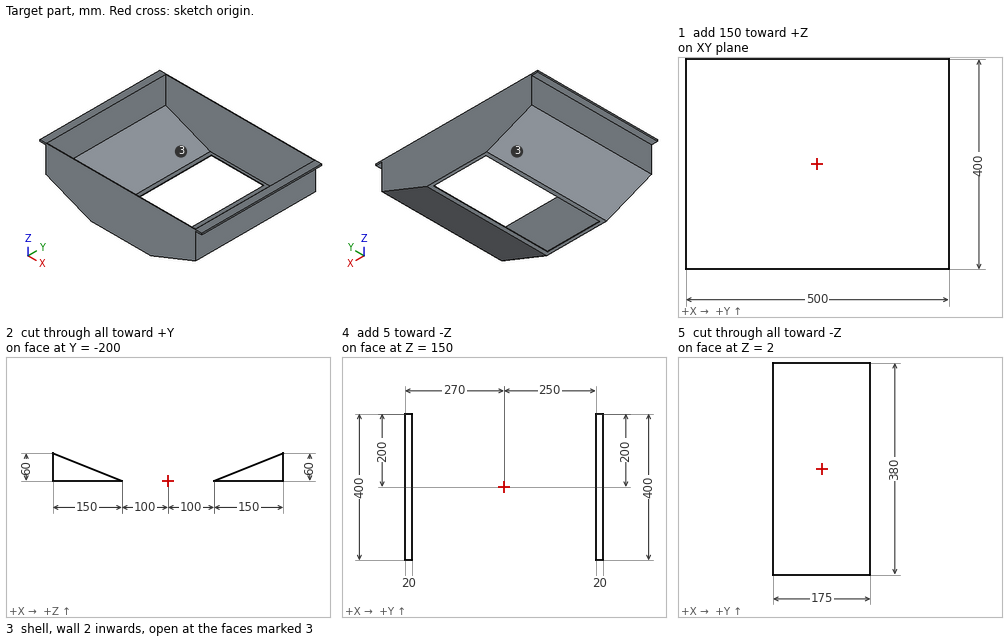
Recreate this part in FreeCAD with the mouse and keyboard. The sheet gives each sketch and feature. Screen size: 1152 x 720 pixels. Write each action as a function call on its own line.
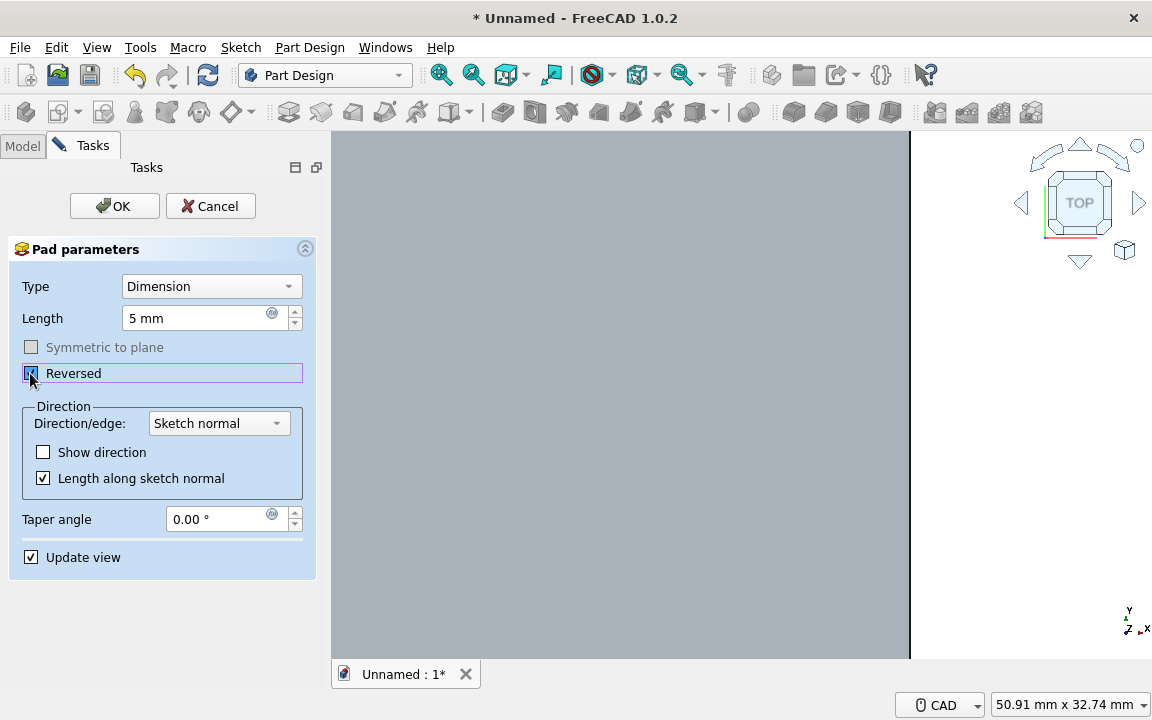
click(115, 206)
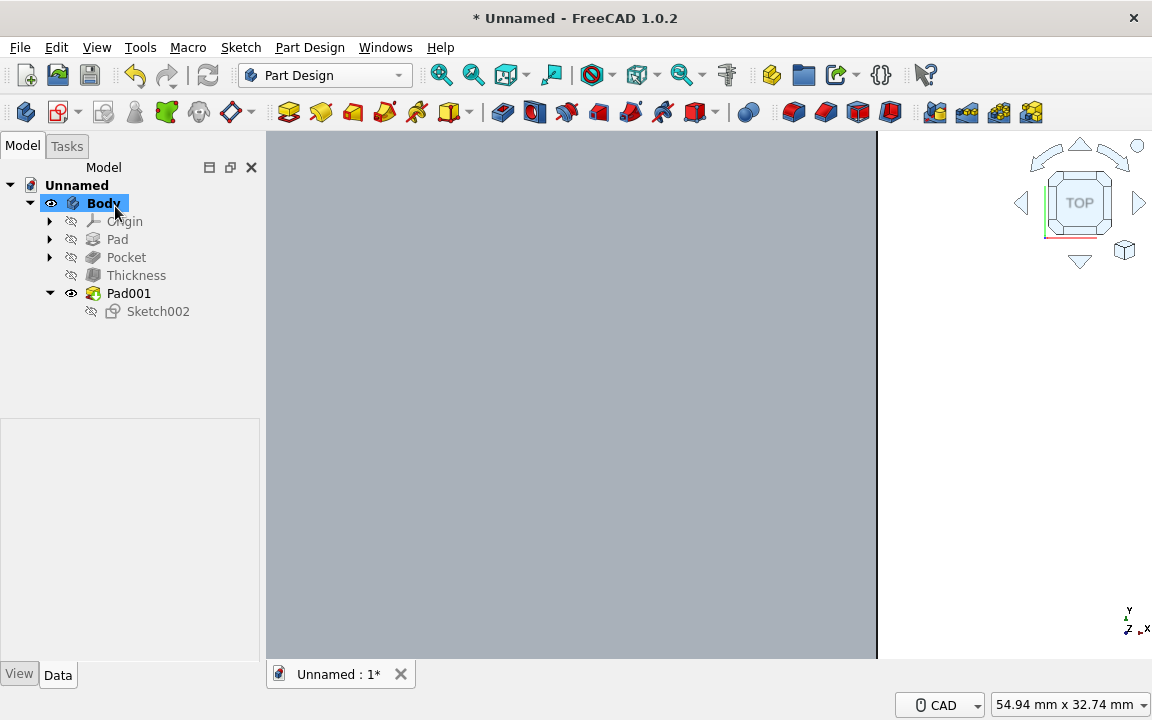
key(v)
key(f)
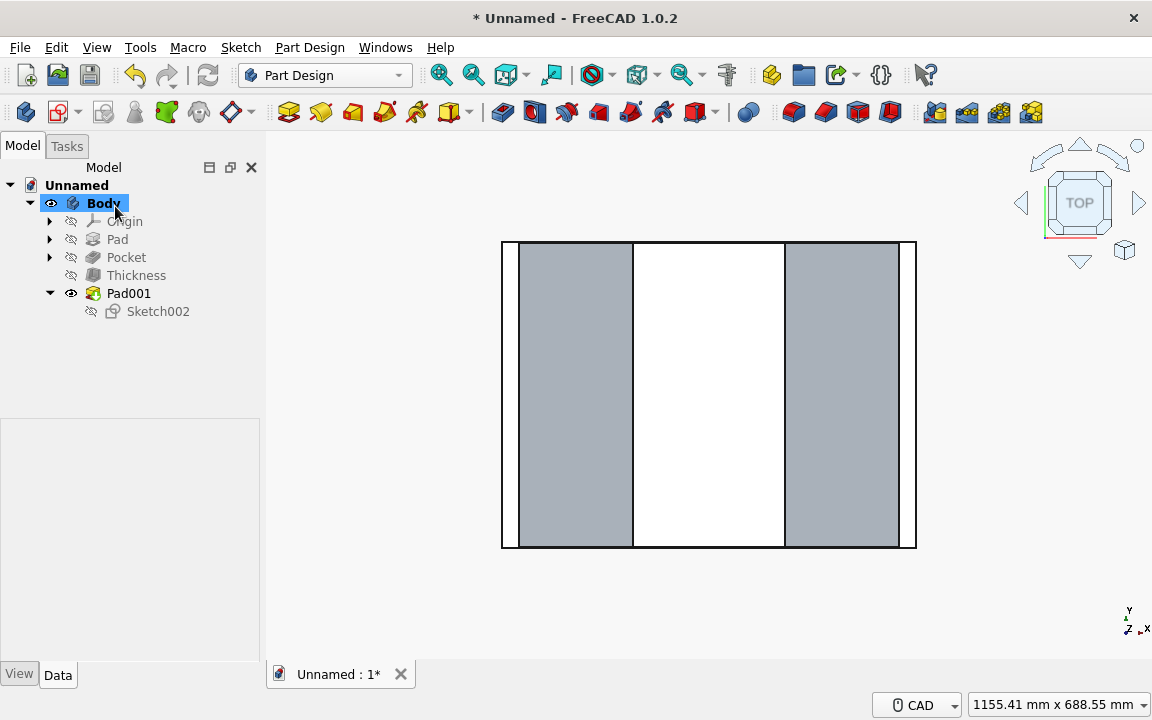
click(709, 351)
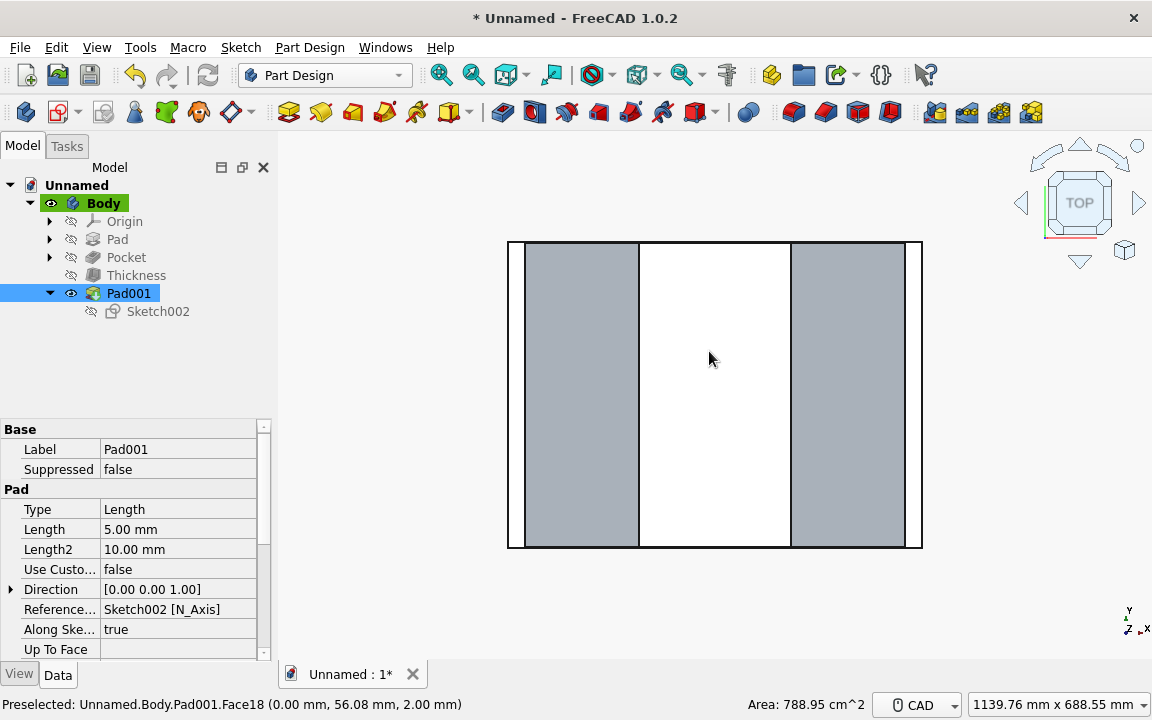
click(58, 112)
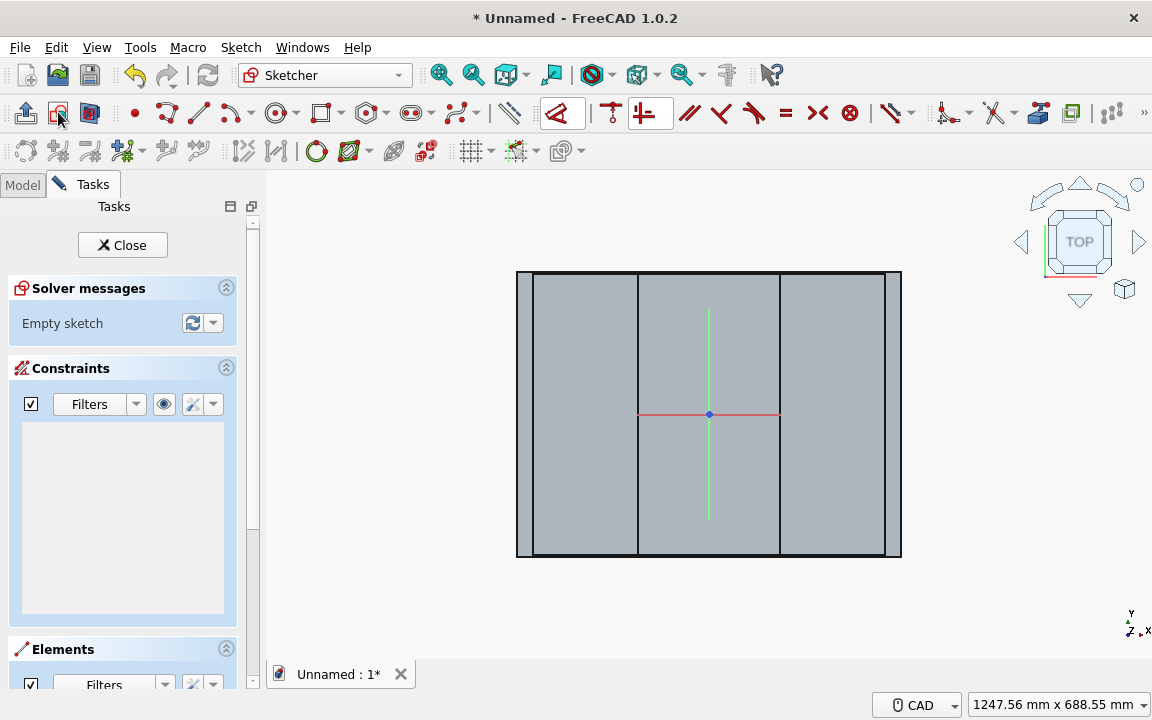
key(g)
key(v)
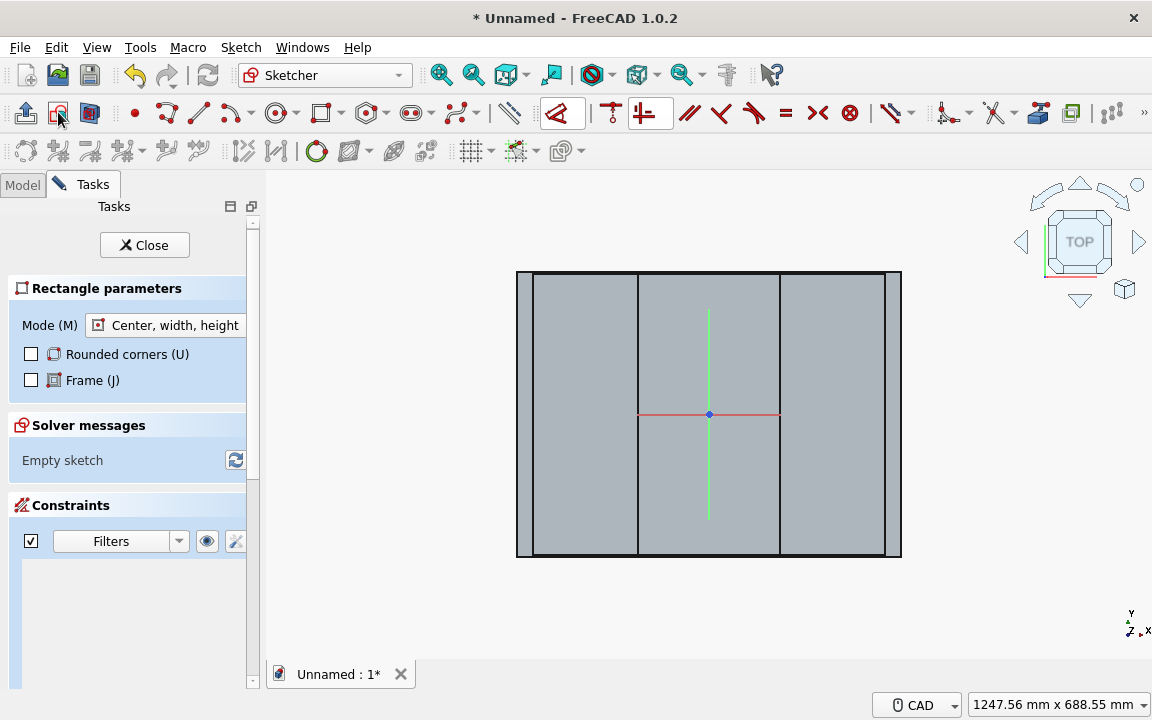
click(709, 414)
click(771, 280)
key(Escape)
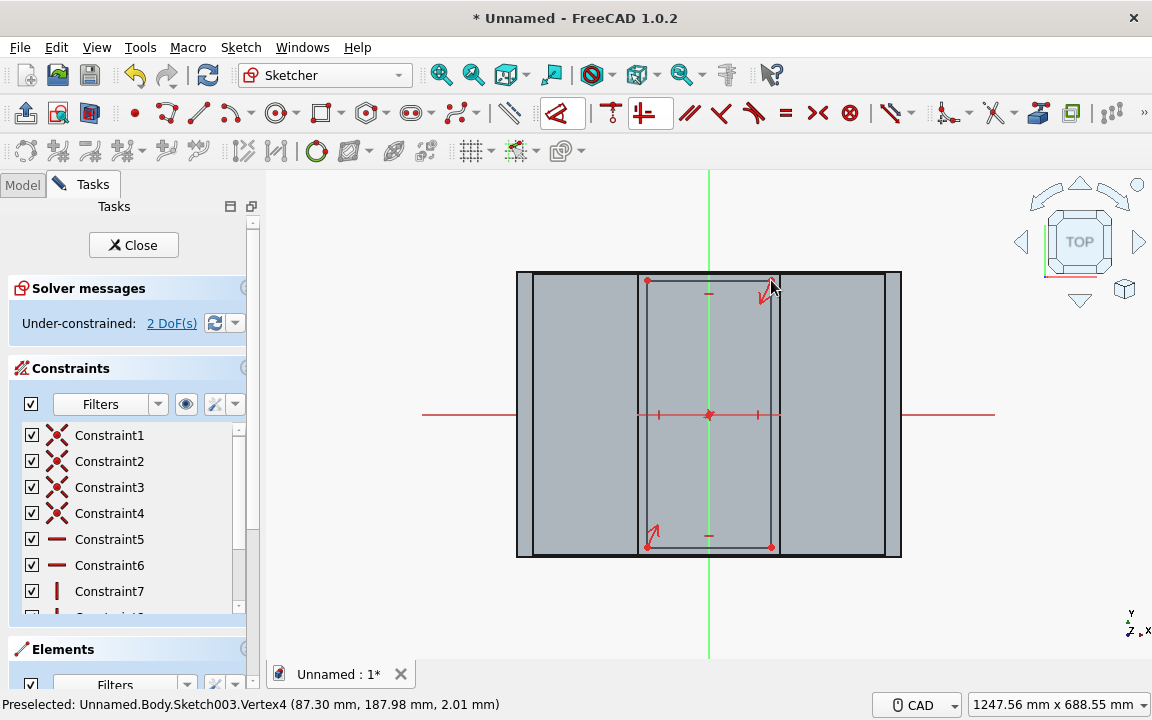
click(684, 548)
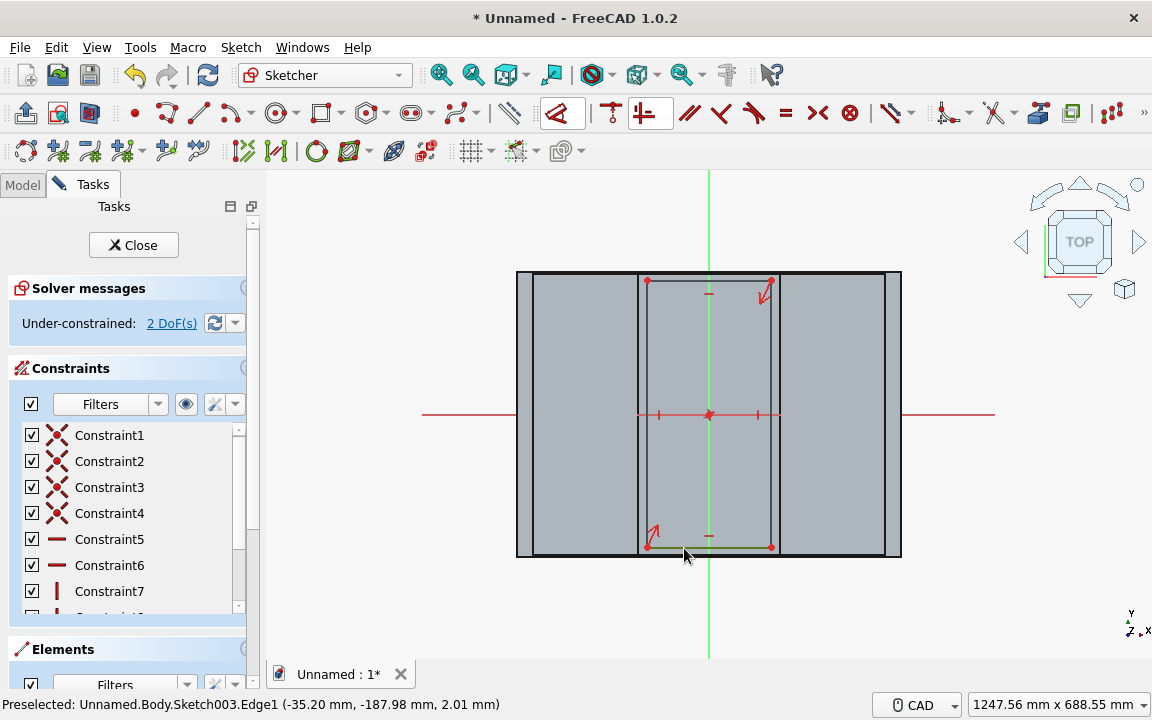
key(l)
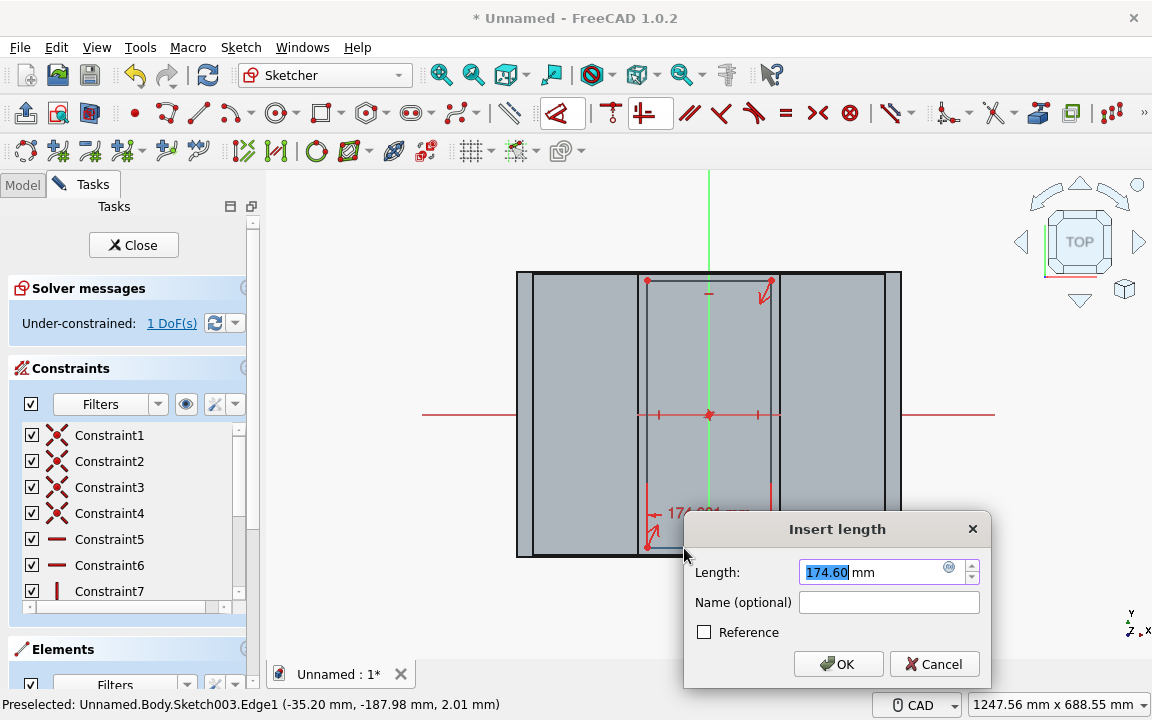
text(175)
key(Return)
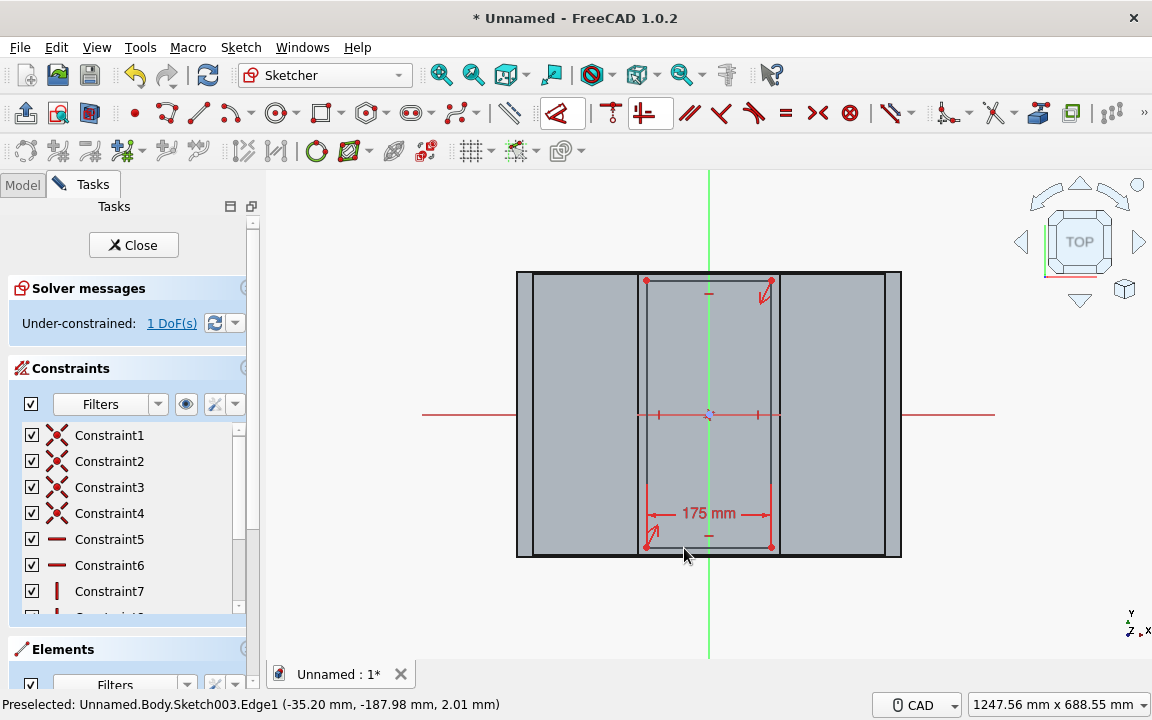
click(771, 468)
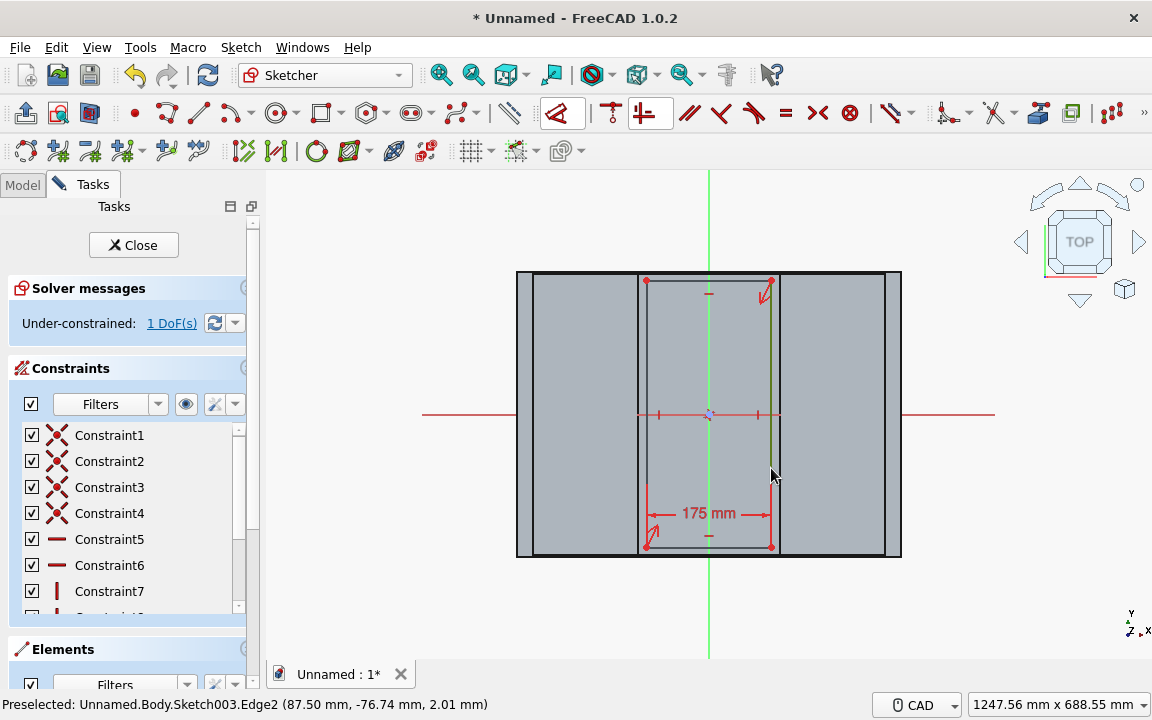
key(i)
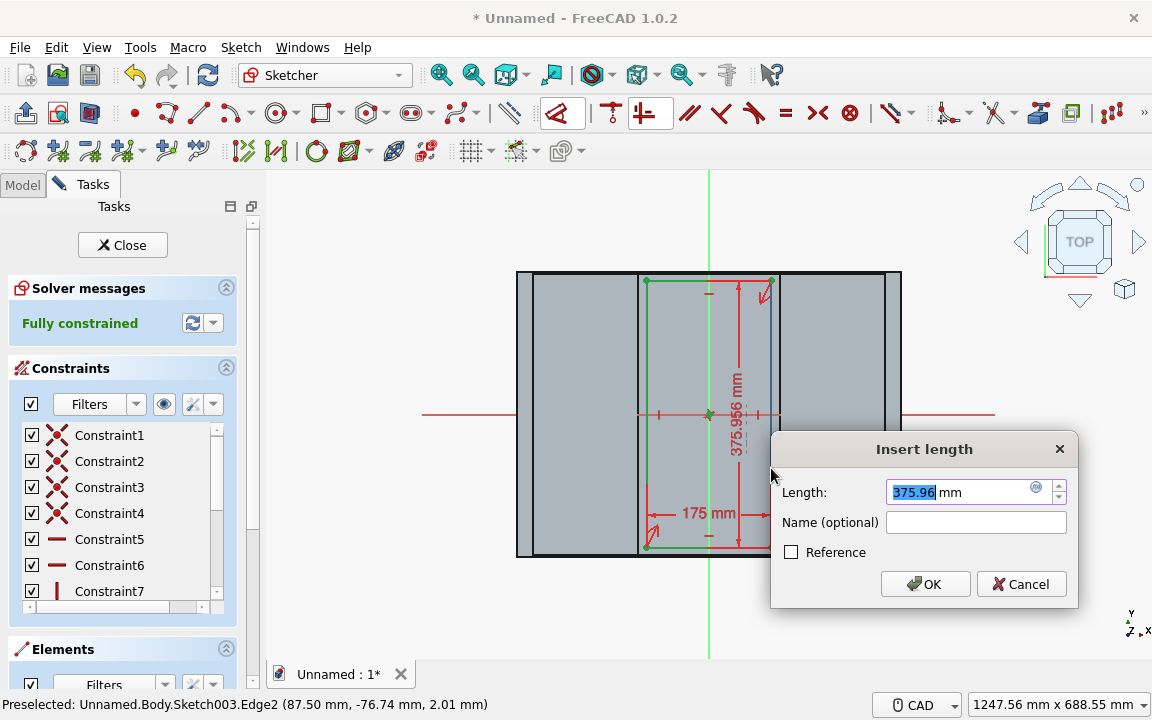
text(380)
key(Return)